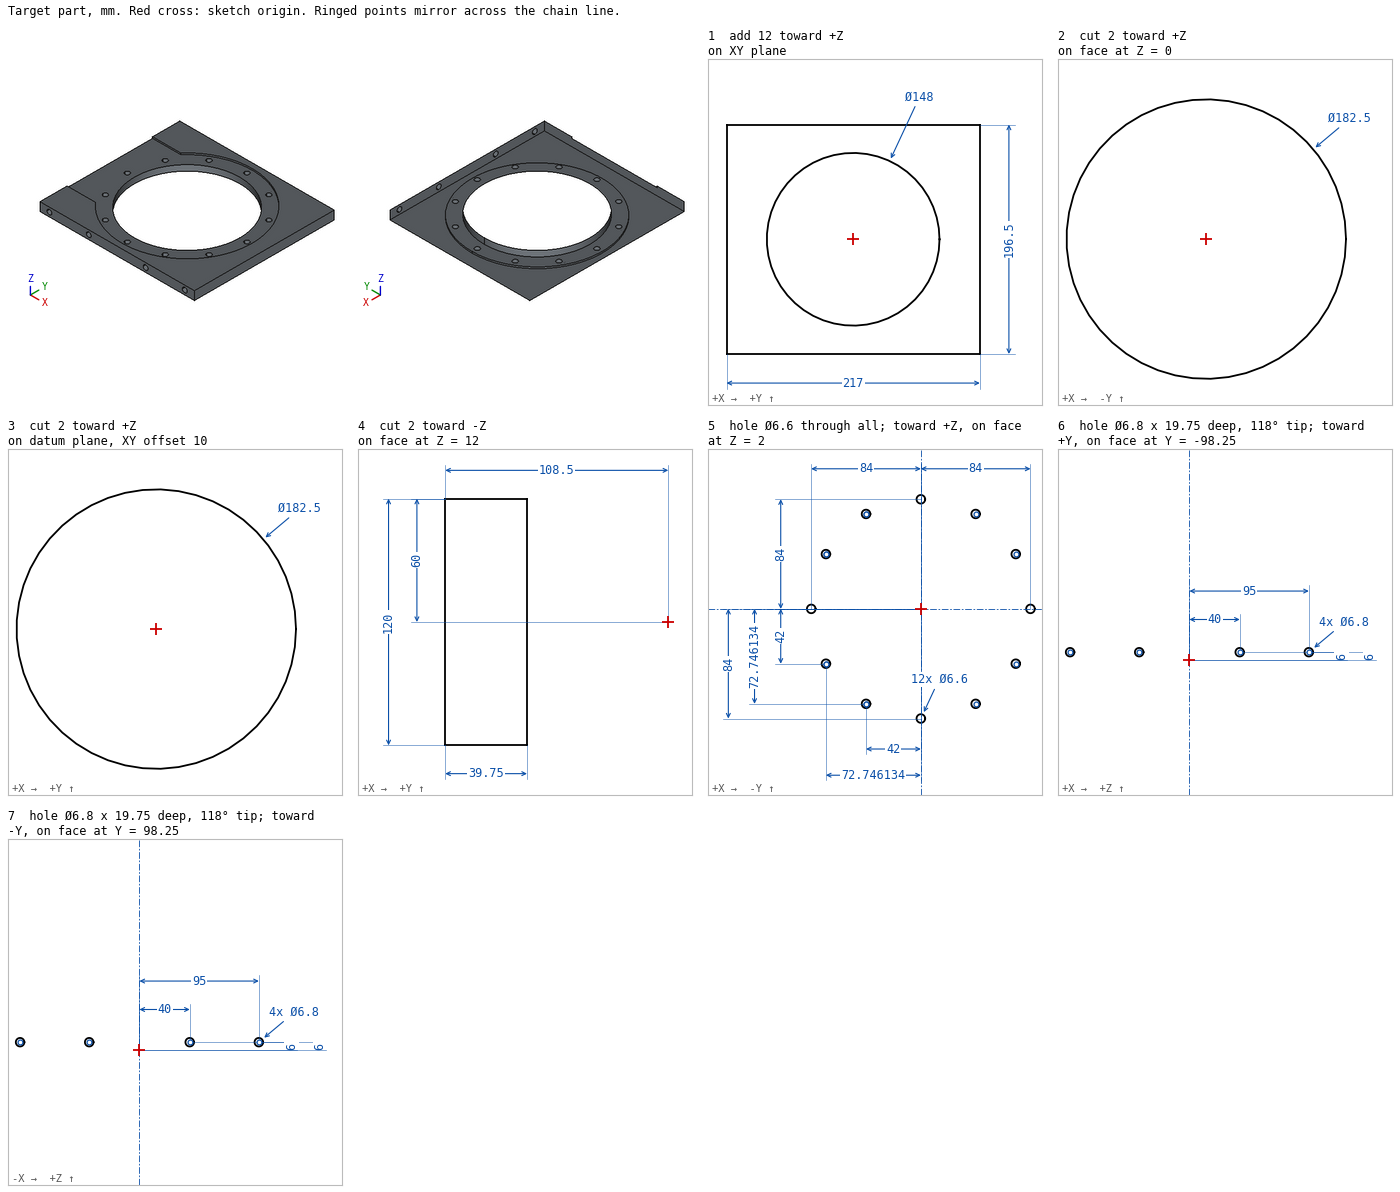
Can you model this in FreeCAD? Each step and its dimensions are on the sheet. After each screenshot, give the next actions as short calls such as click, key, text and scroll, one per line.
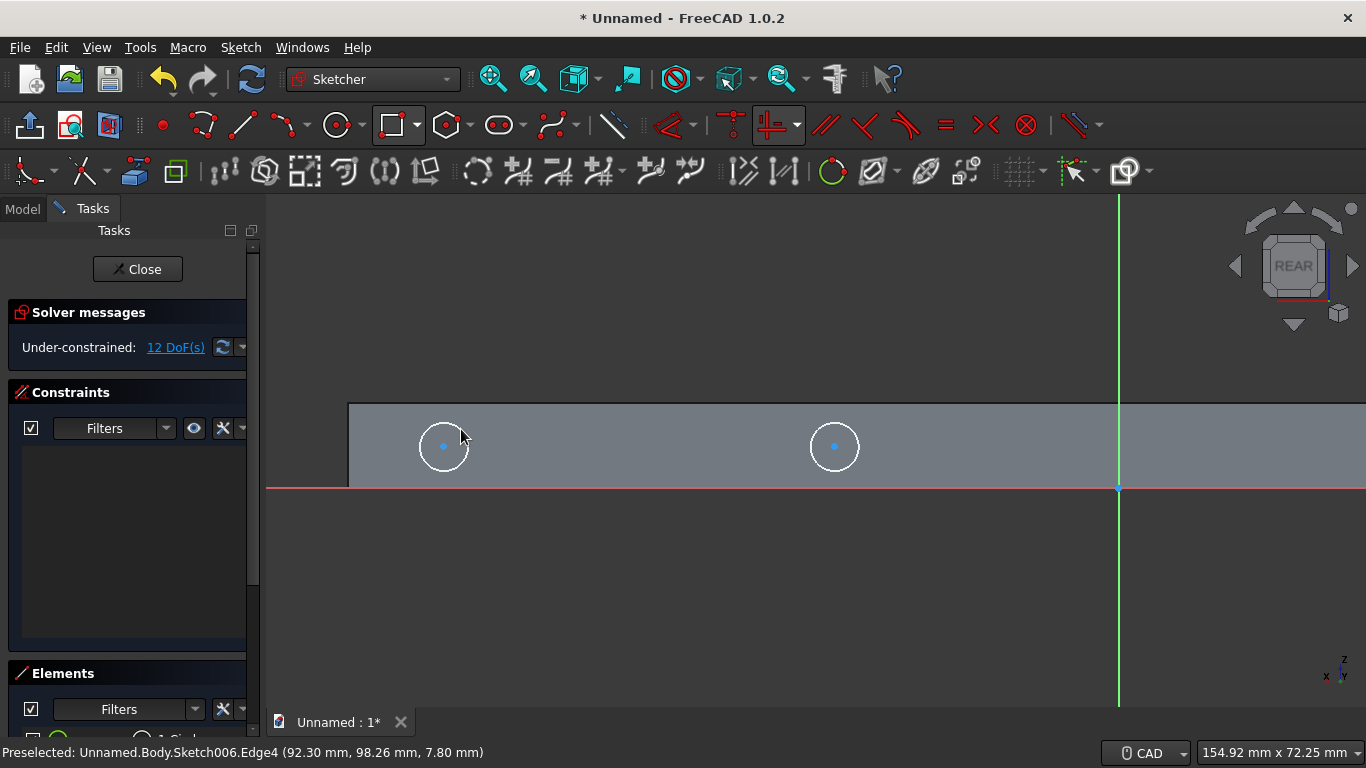
scroll(445, 447, down, 4)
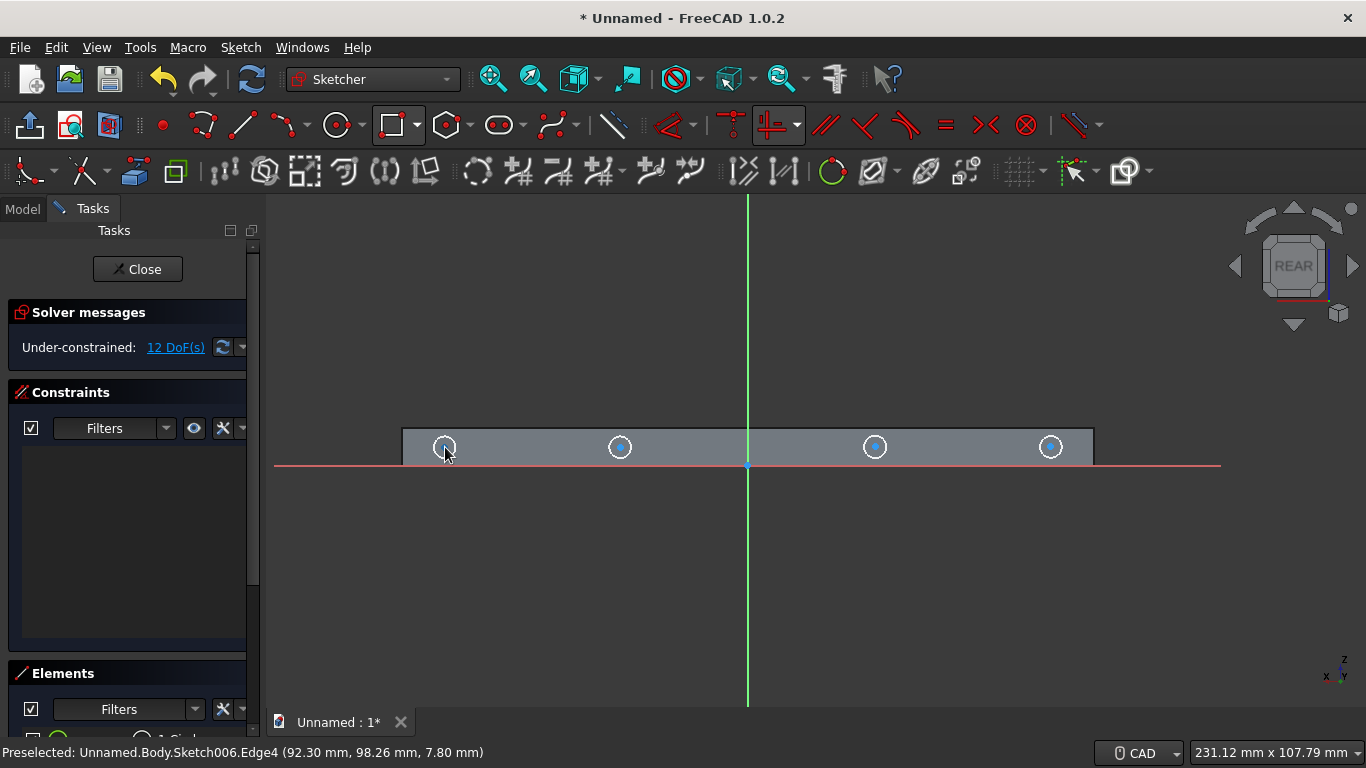
scroll(1059, 439, up, 2)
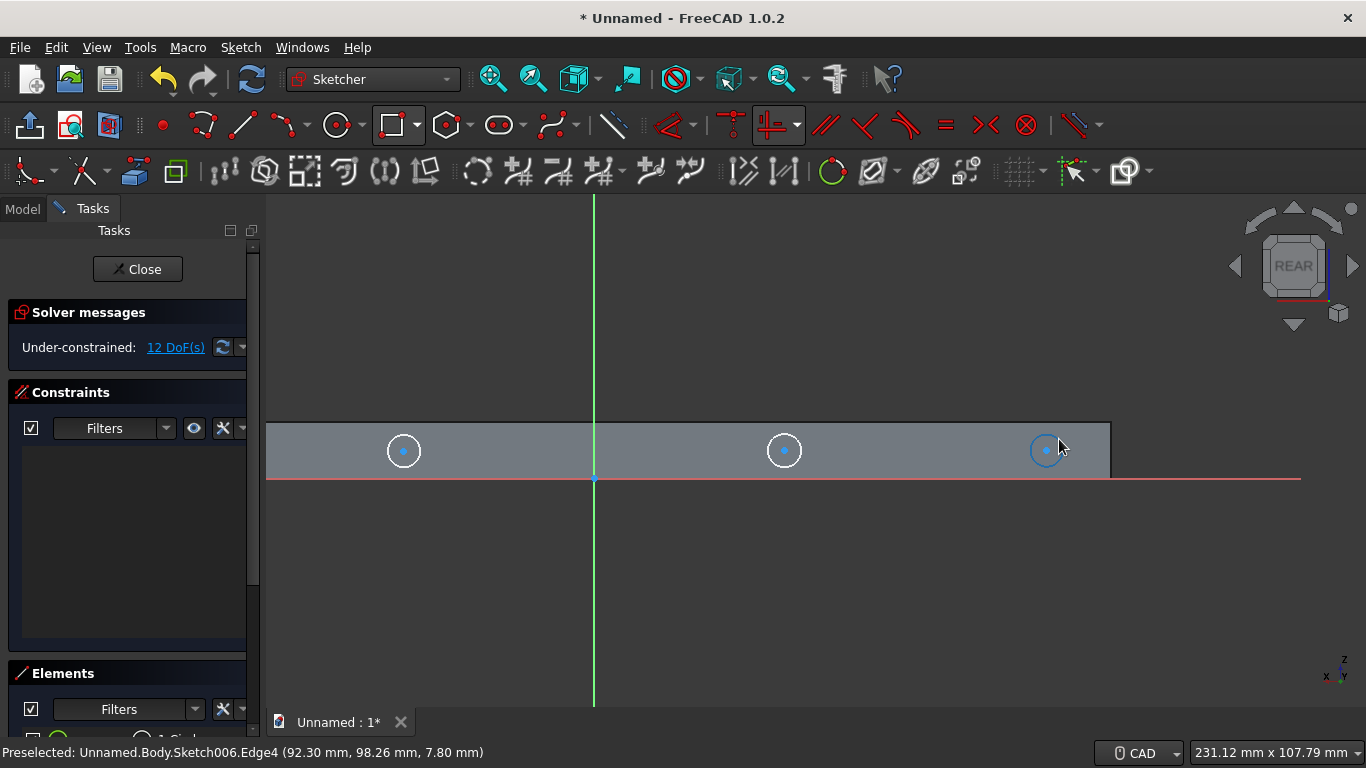
click(1058, 439)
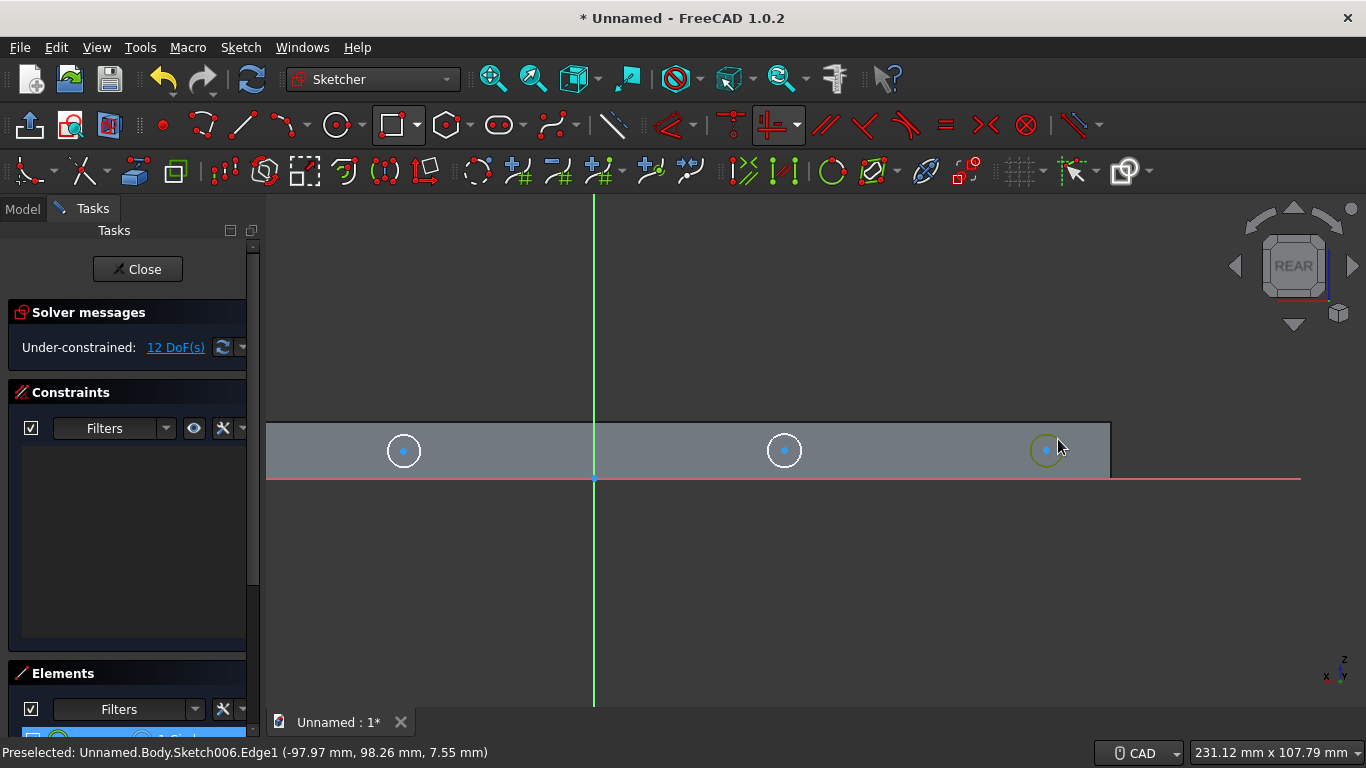
click(796, 439)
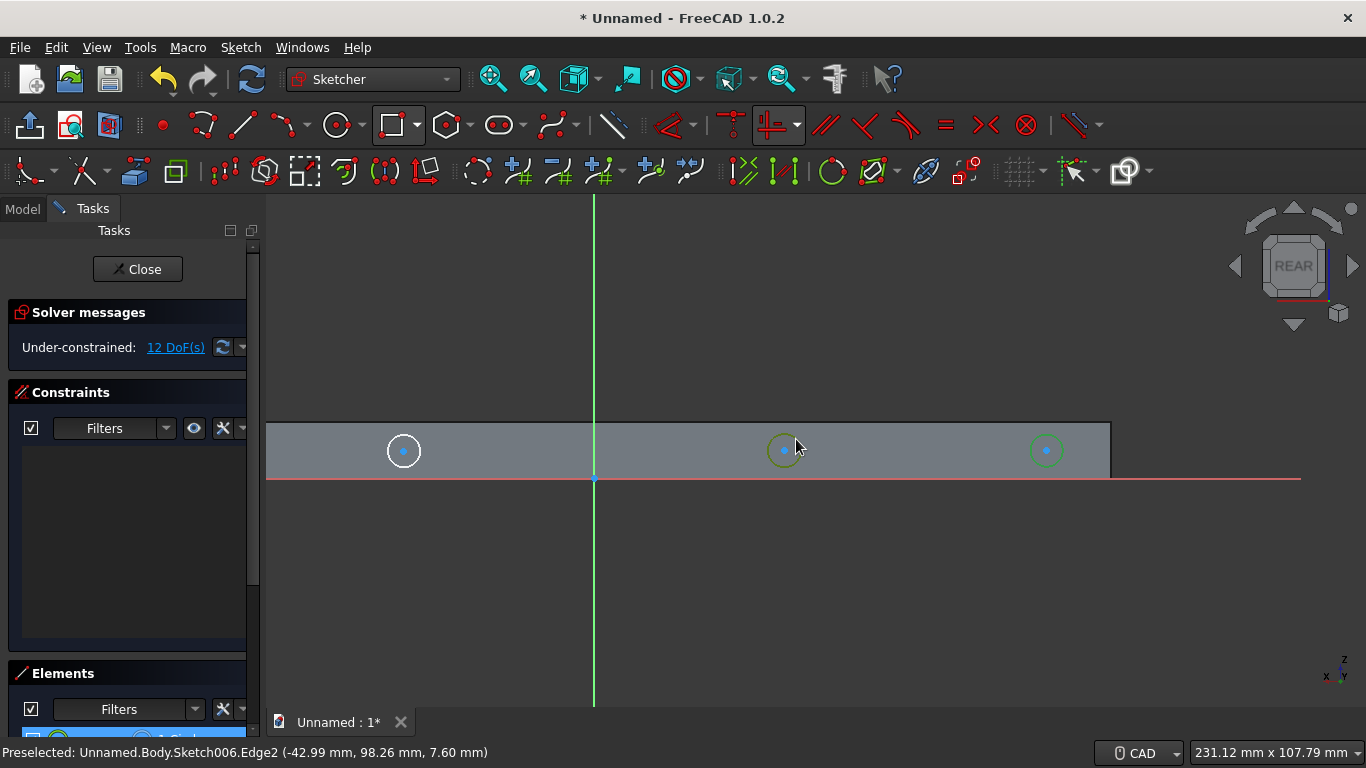
click(415, 440)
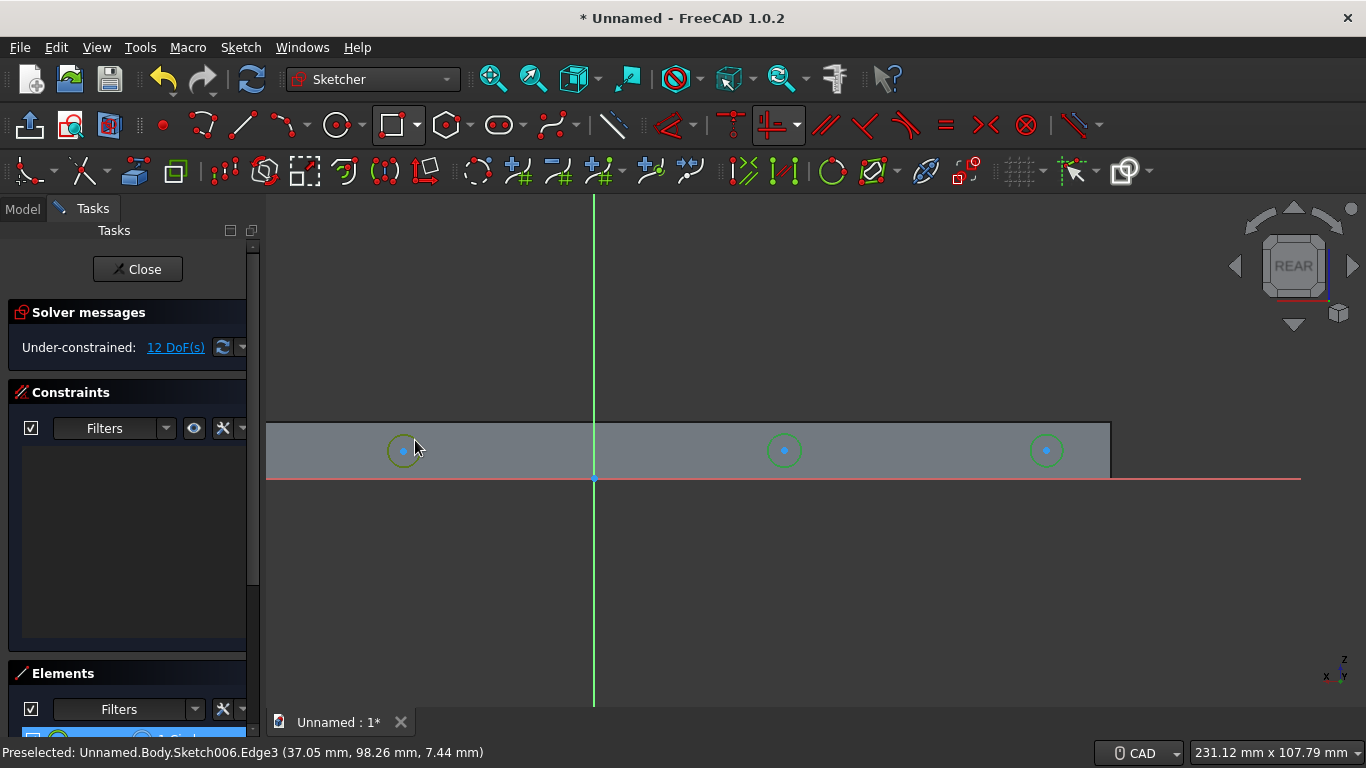
scroll(1059, 439, down, 2)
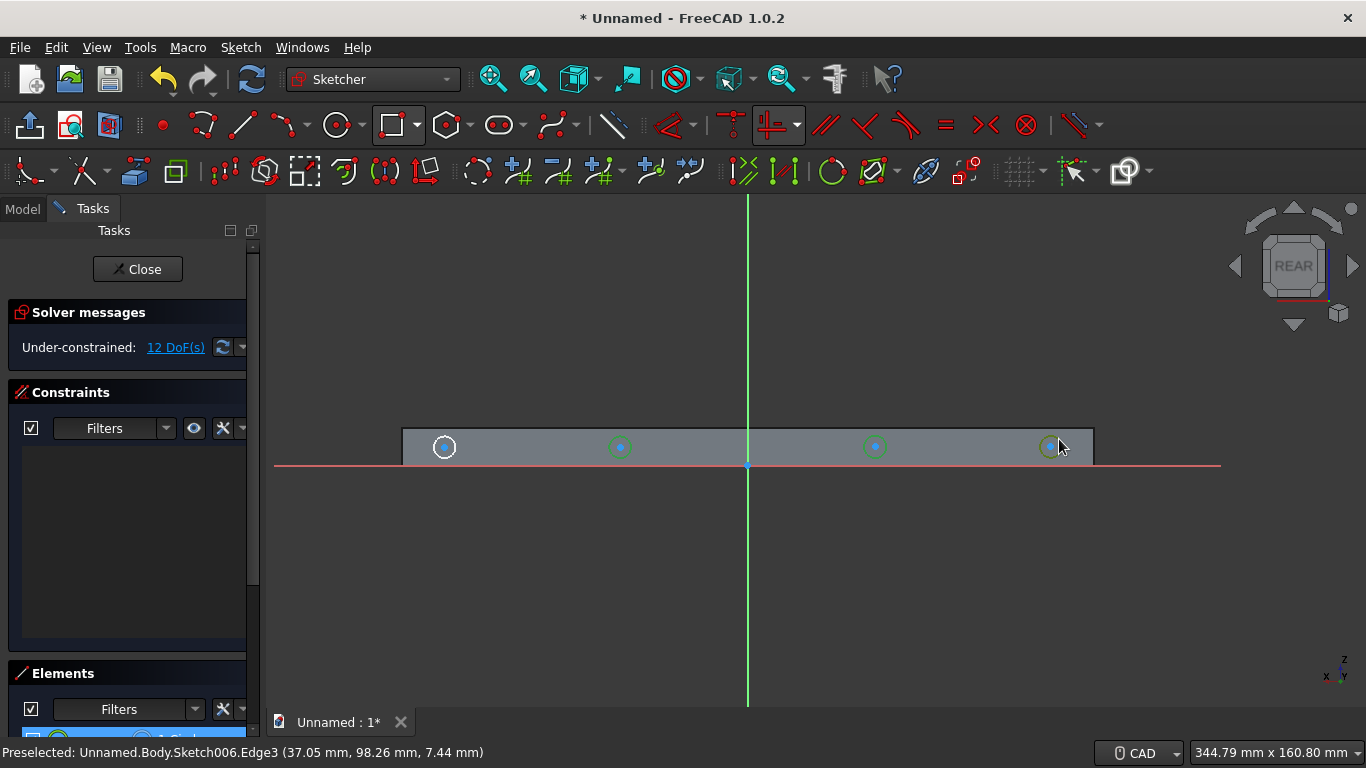
scroll(452, 440, up, 2)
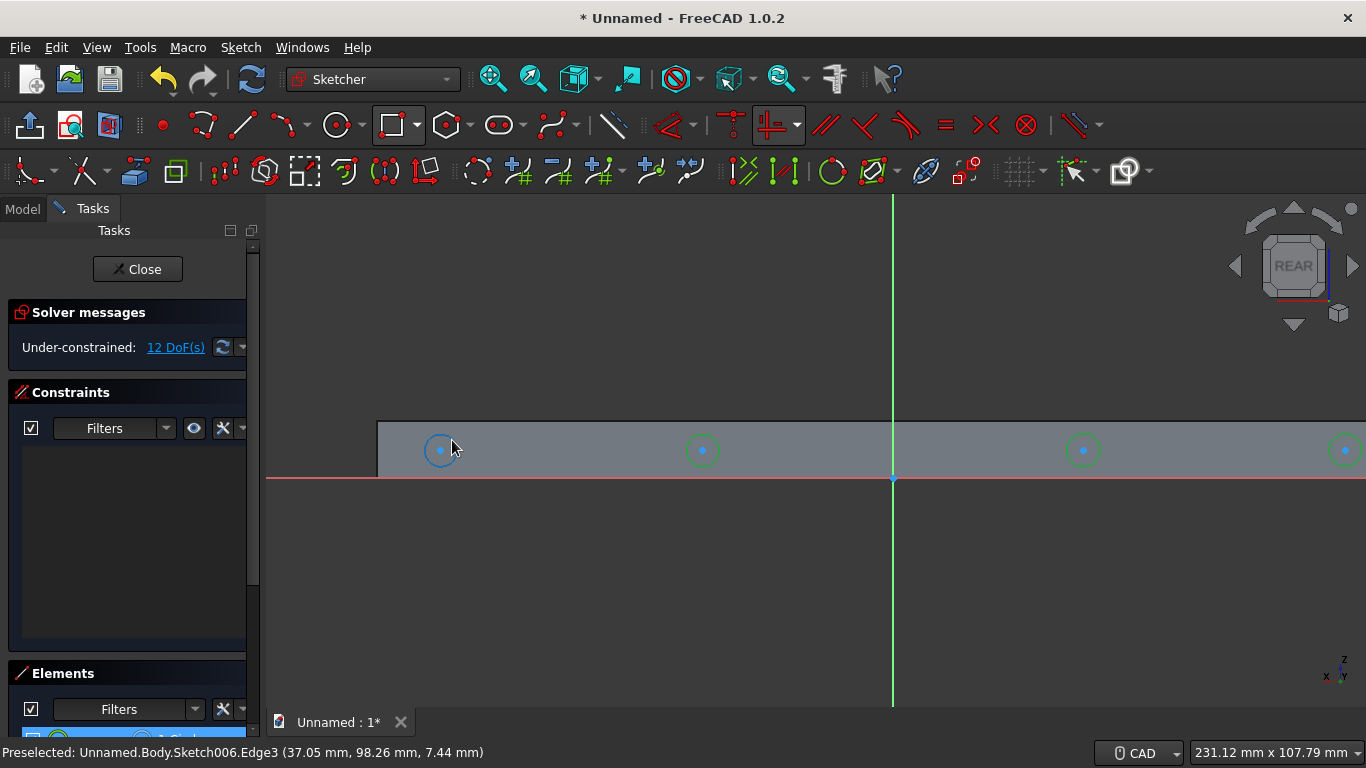
click(452, 439)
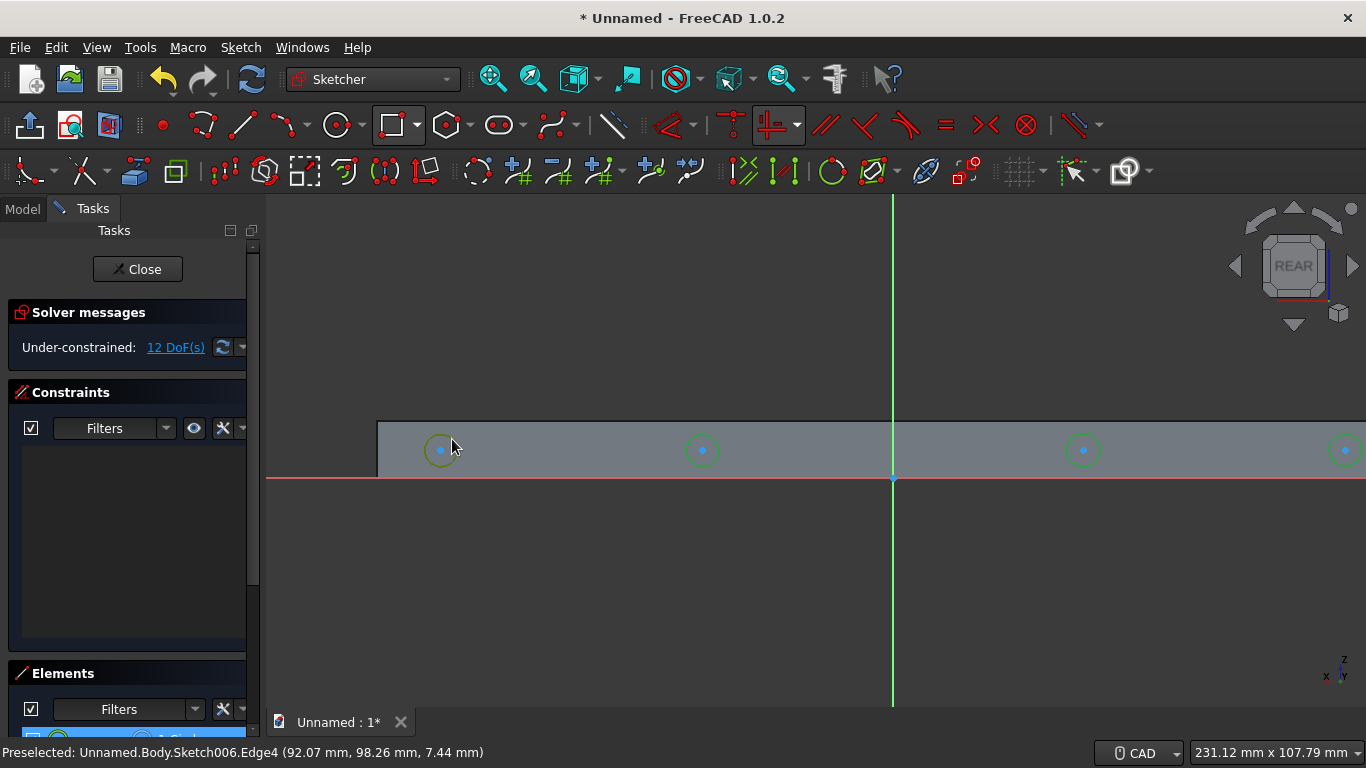
click(946, 126)